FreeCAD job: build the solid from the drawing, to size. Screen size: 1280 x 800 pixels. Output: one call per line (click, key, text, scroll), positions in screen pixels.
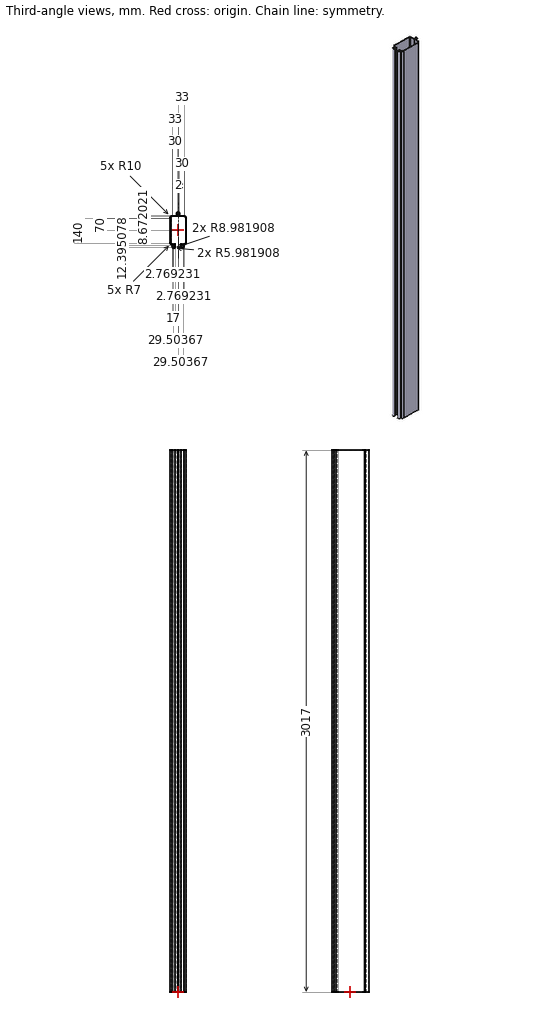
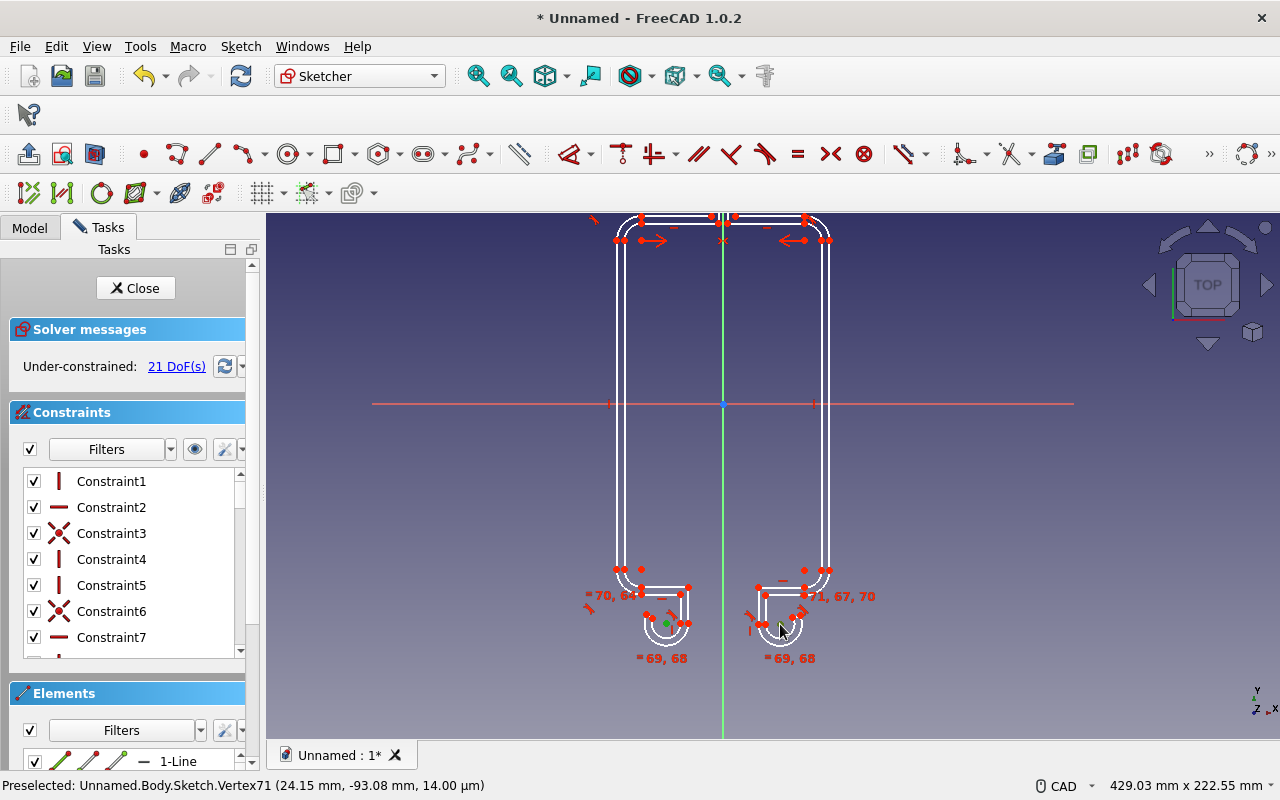
click(723, 677)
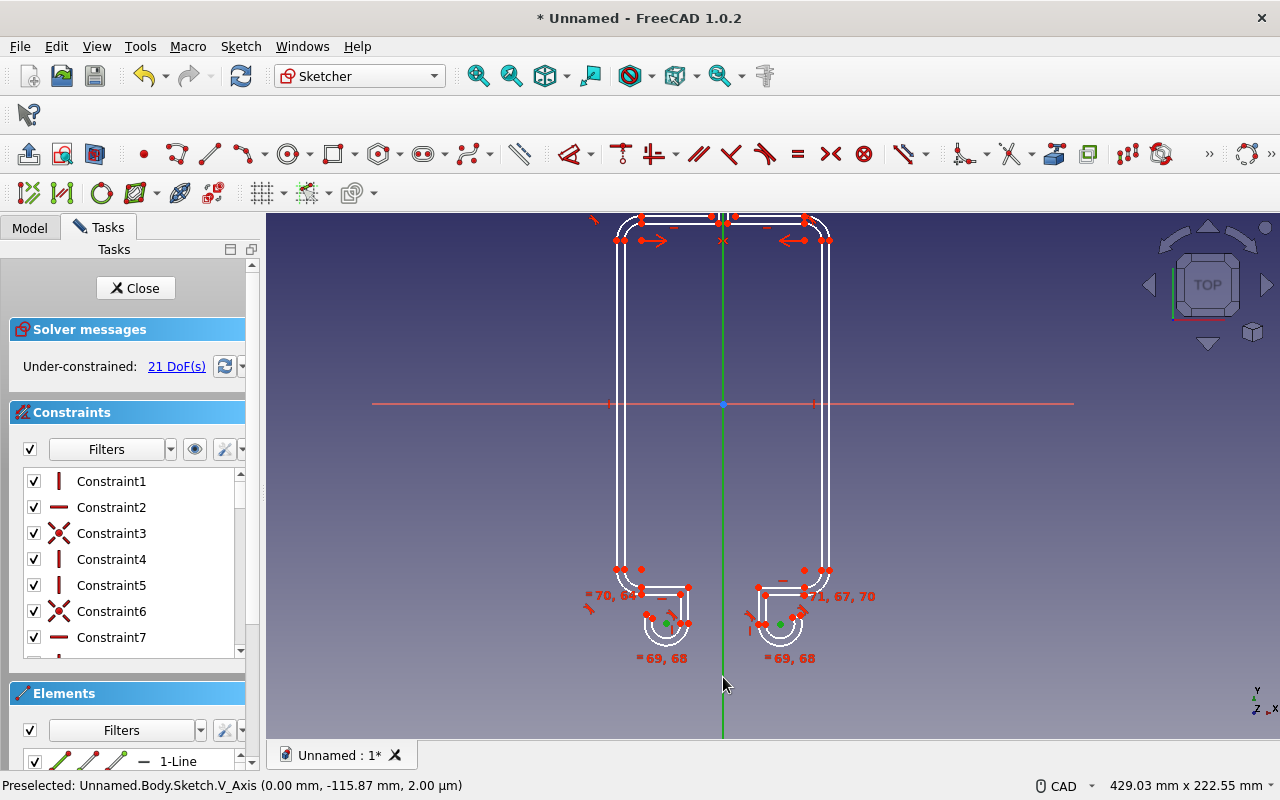
click(831, 154)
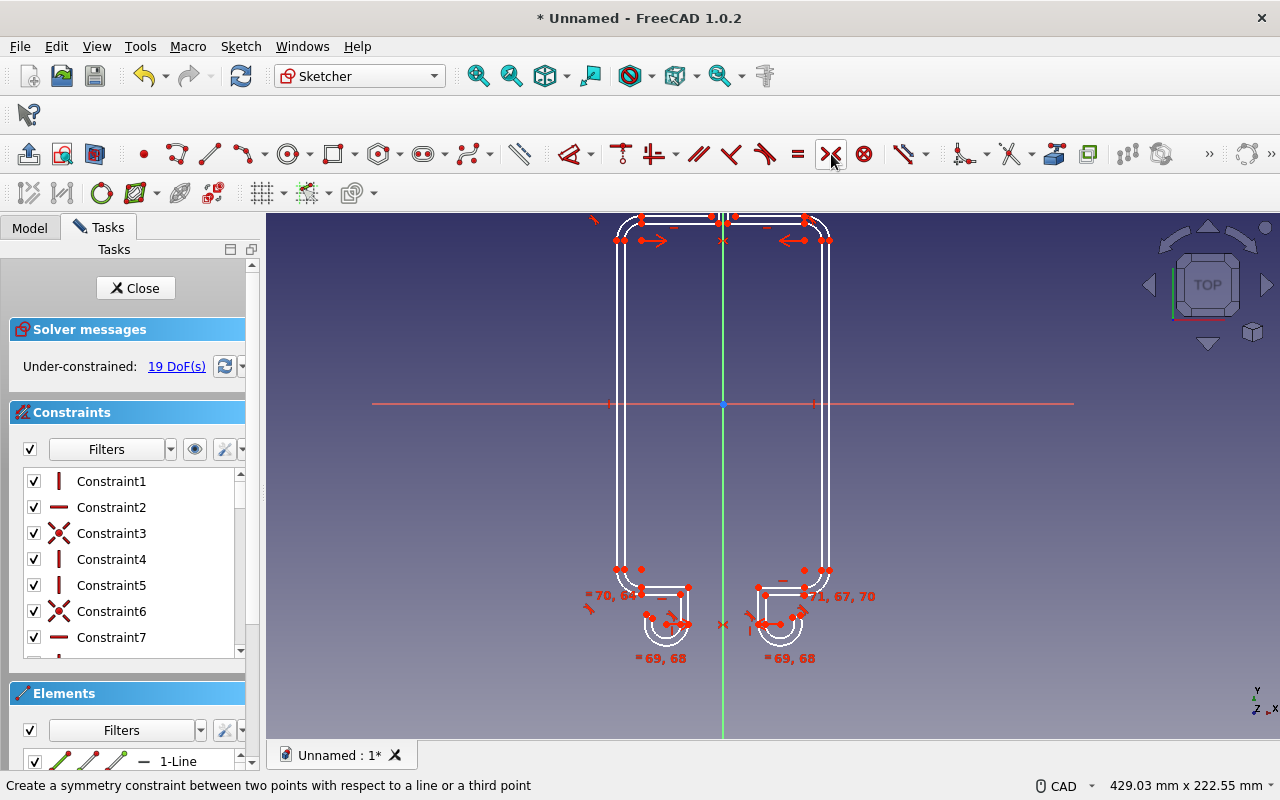
click(568, 154)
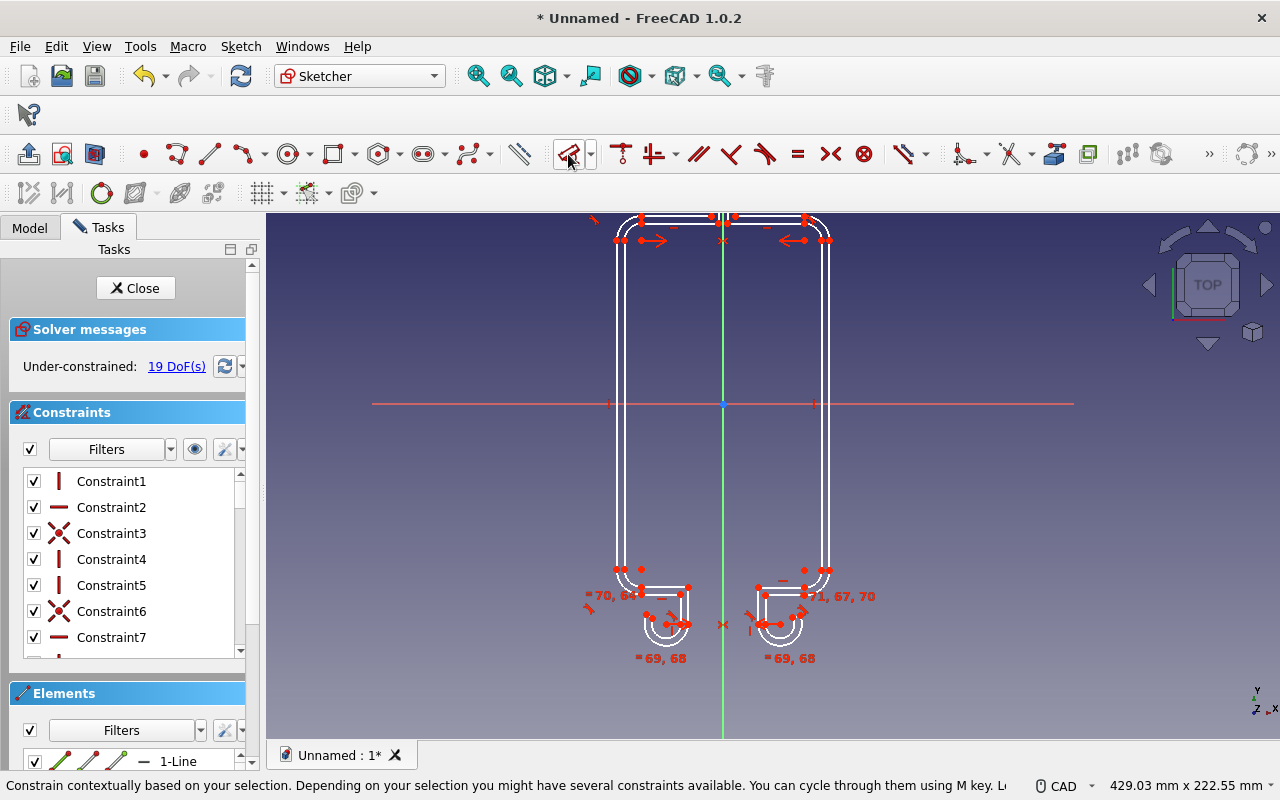
scroll(618, 578, up, 3)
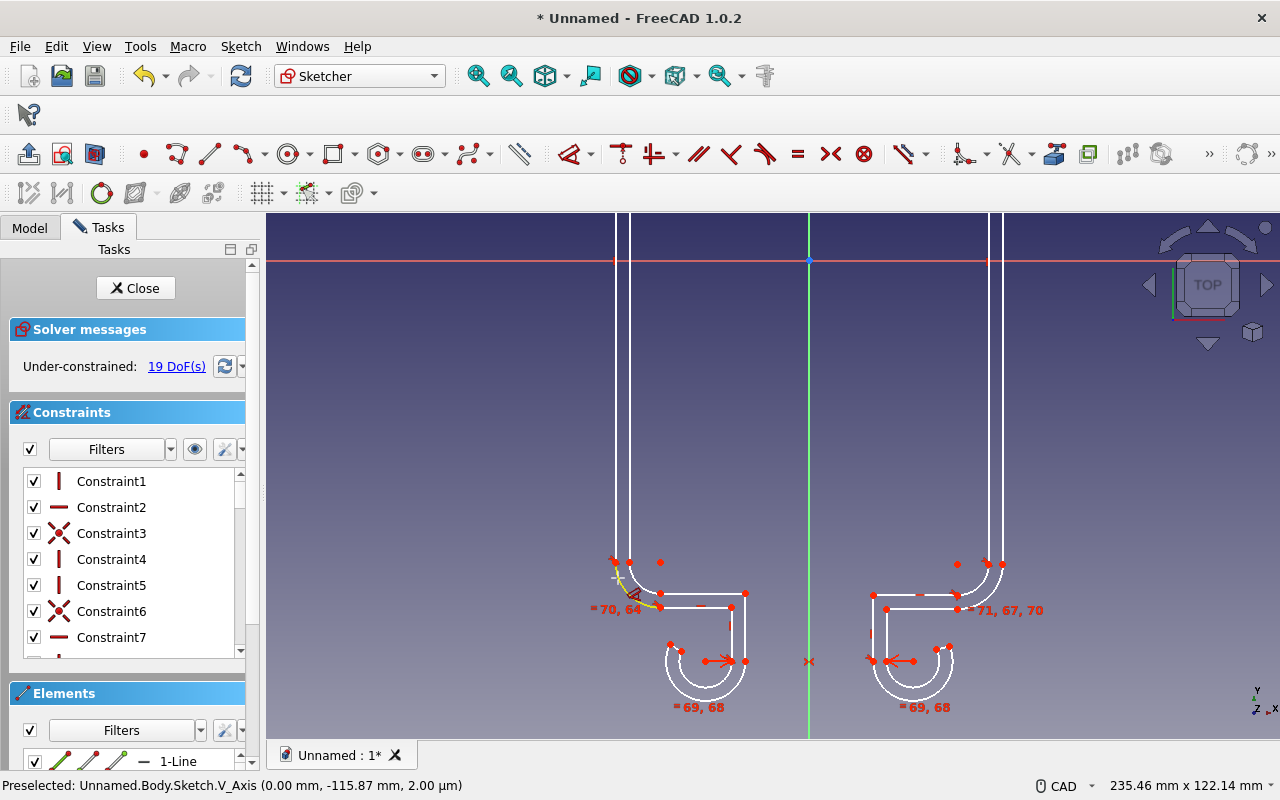
click(618, 577)
click(588, 587)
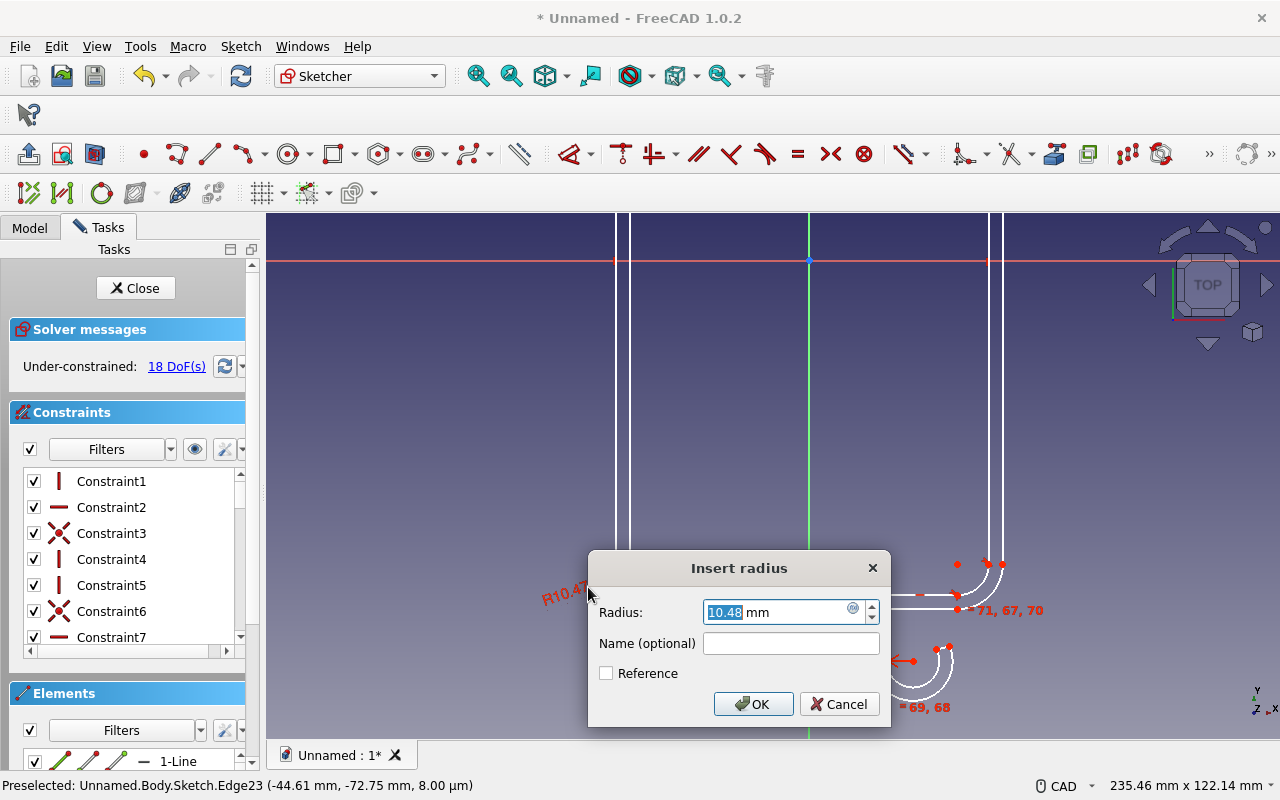
text(10)
key(Return)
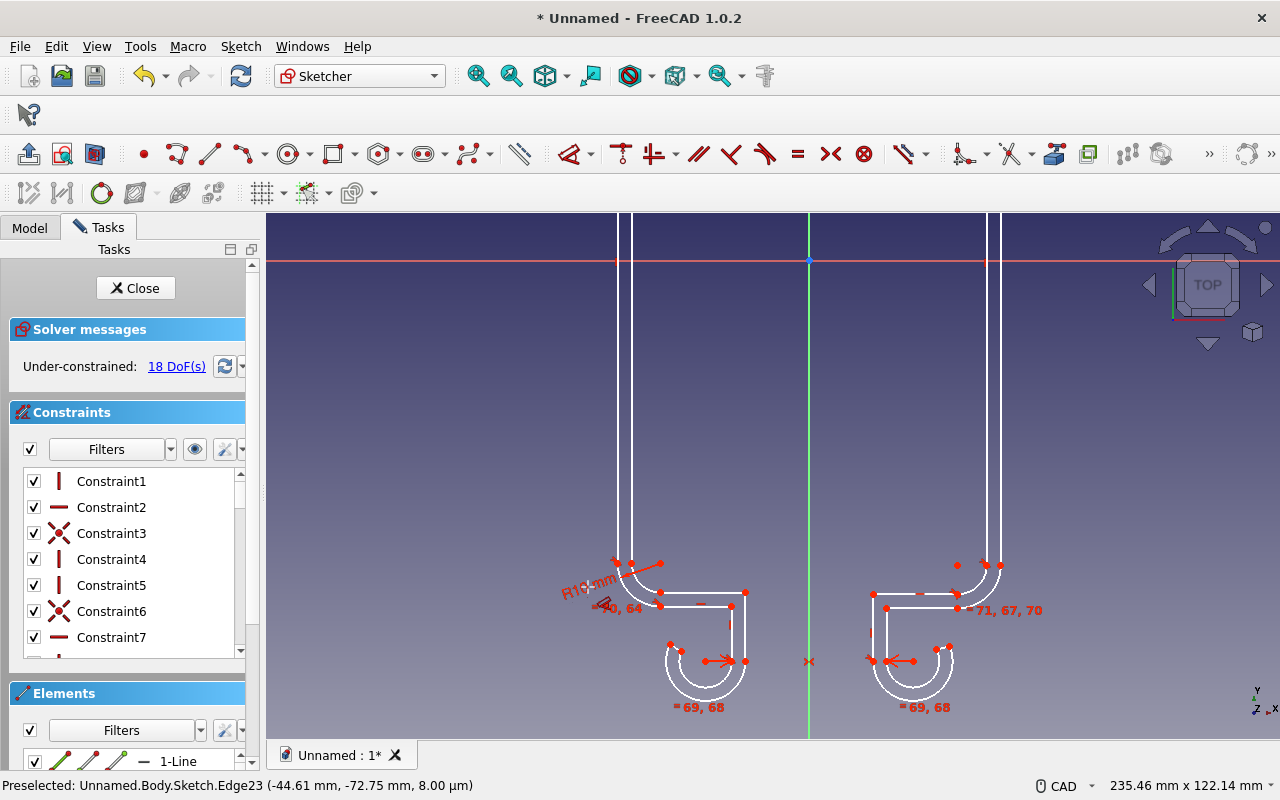
scroll(685, 678, up, 3)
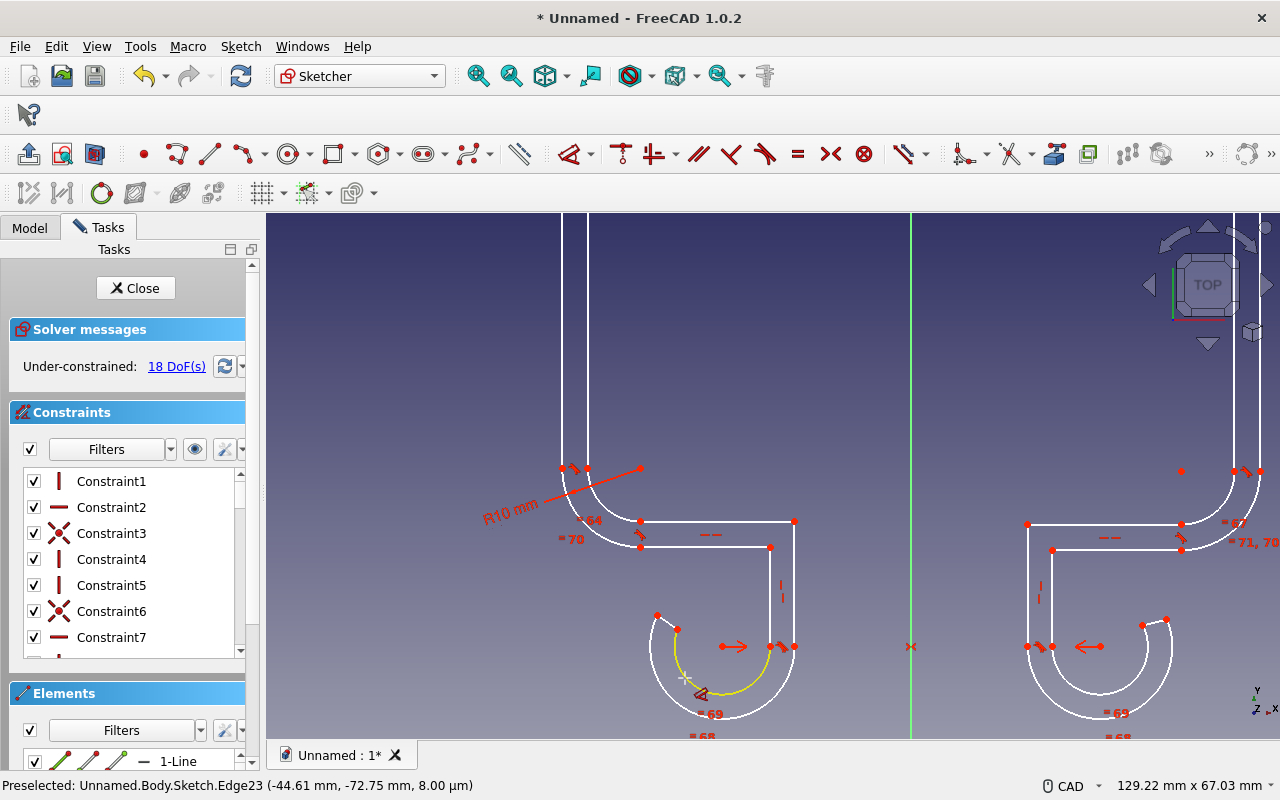
click(685, 677)
click(672, 585)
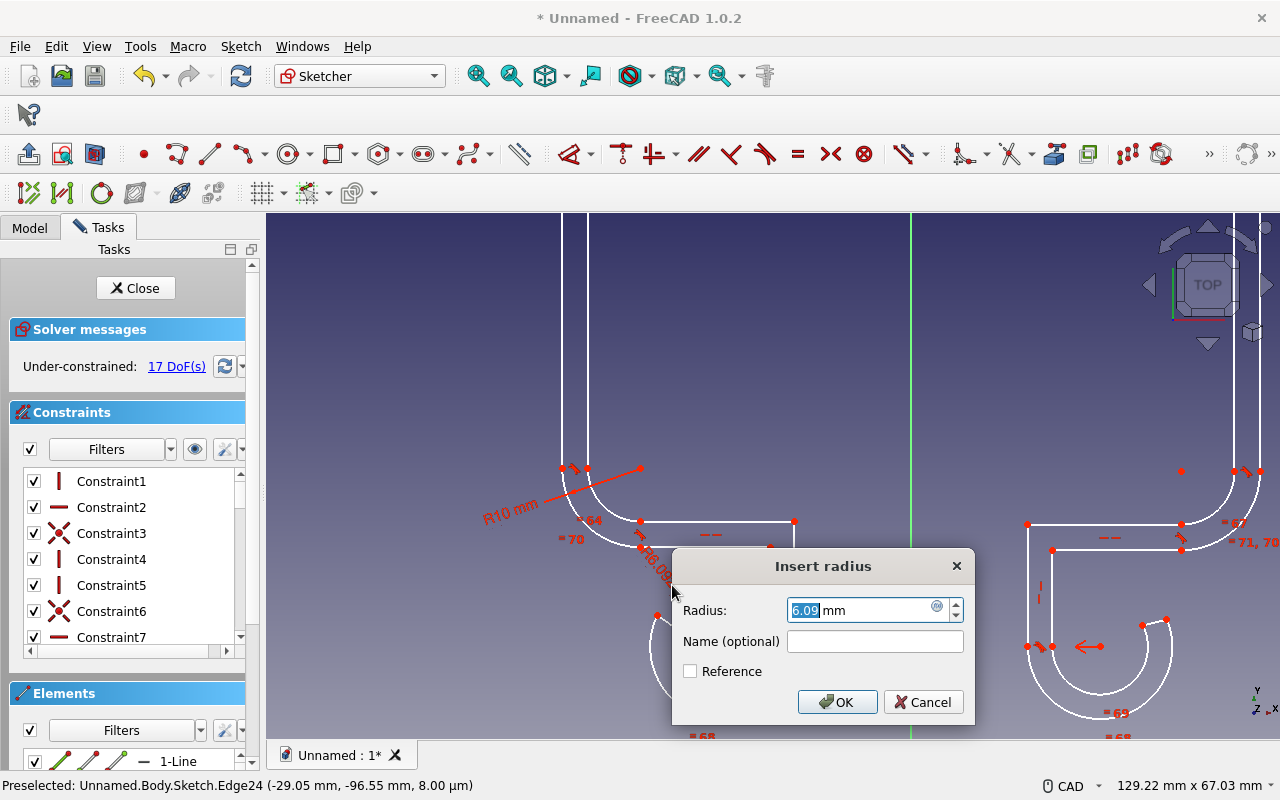
text(5.981908)
key(Return)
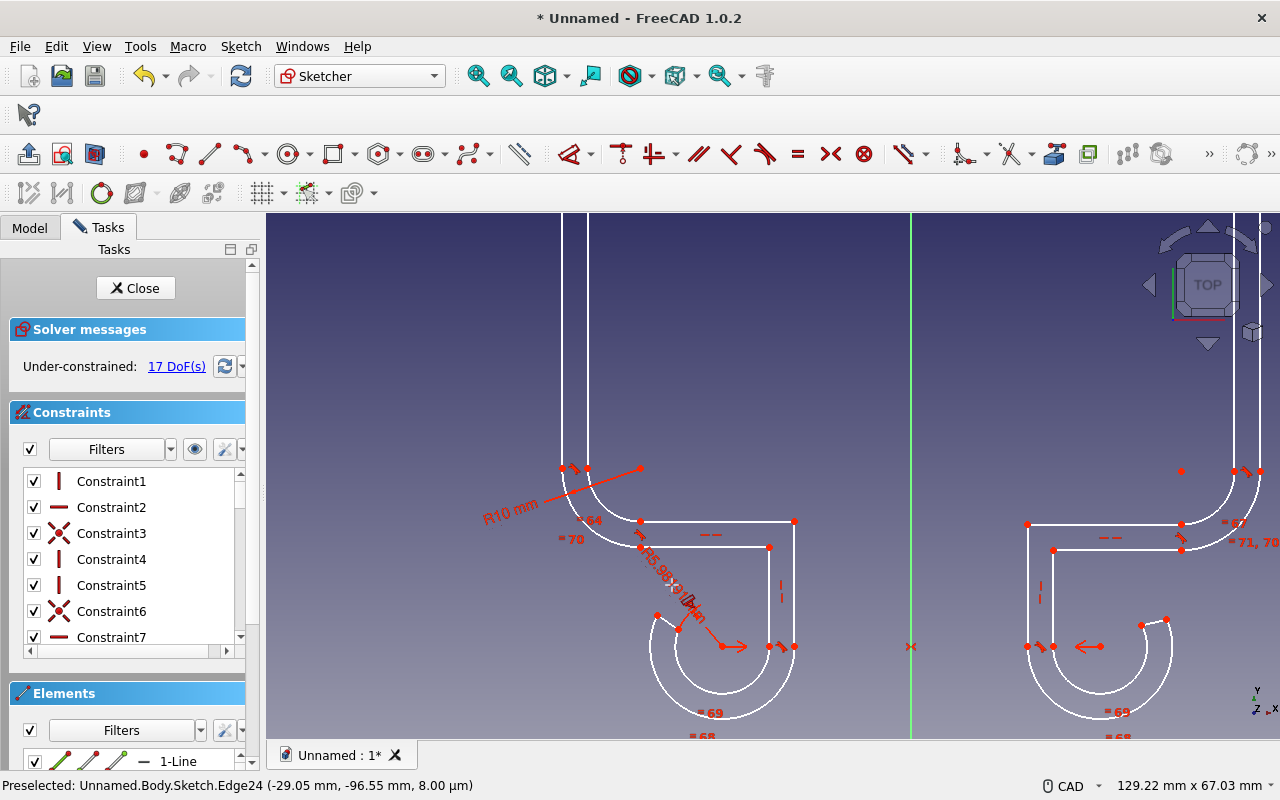
click(664, 689)
click(638, 708)